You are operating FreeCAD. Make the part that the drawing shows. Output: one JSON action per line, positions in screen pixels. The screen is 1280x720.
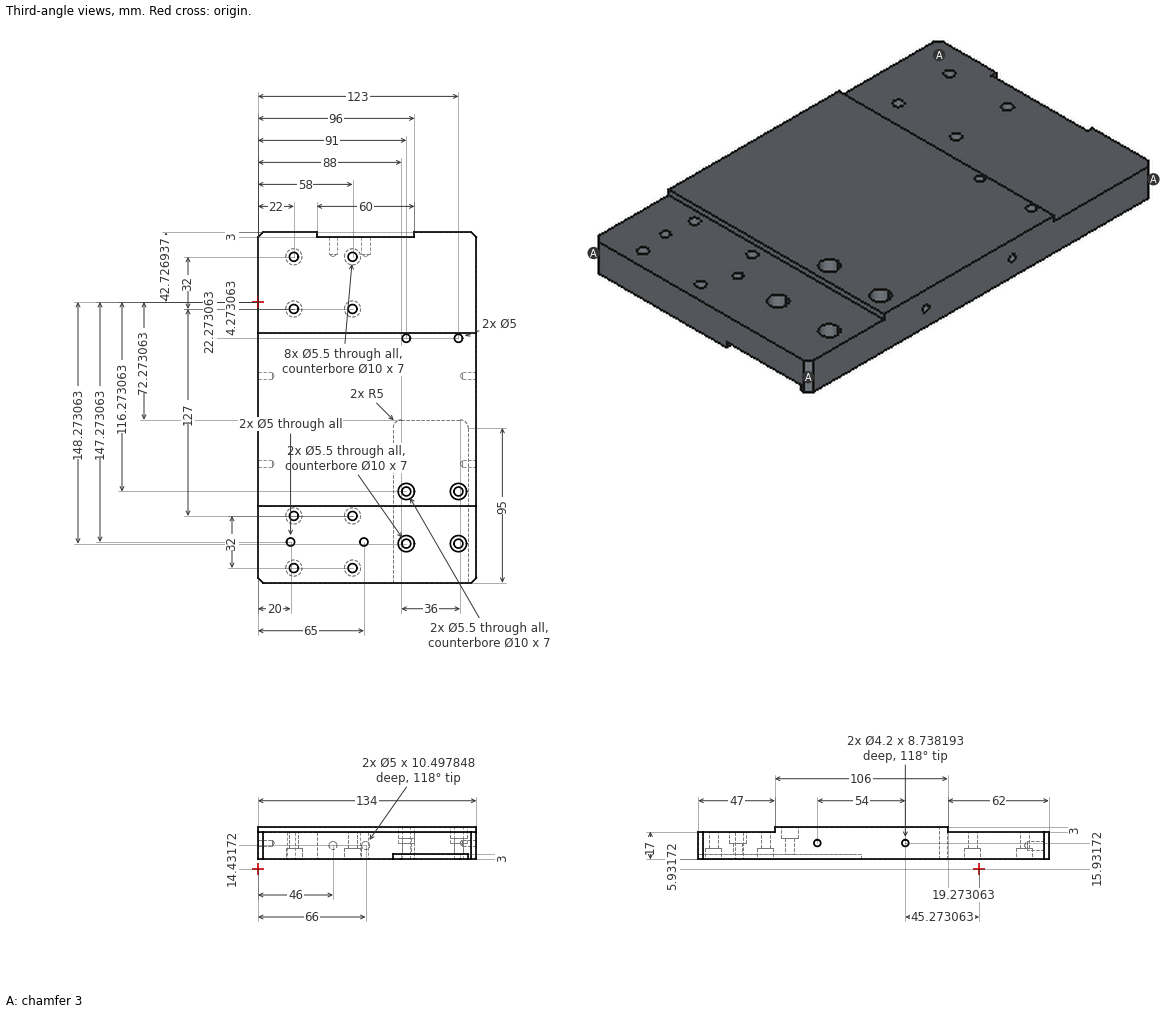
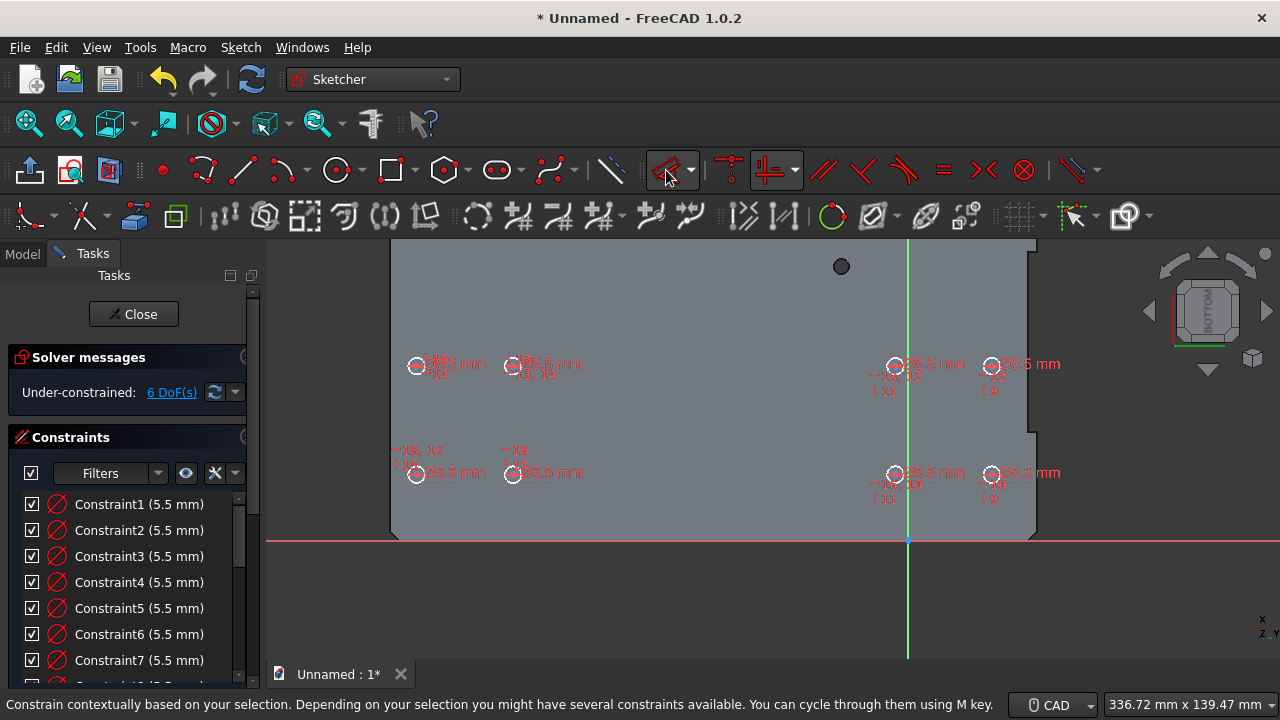
{"action": "left_click", "coordinate": [992, 366]}
{"action": "left_click", "coordinate": [1026, 453]}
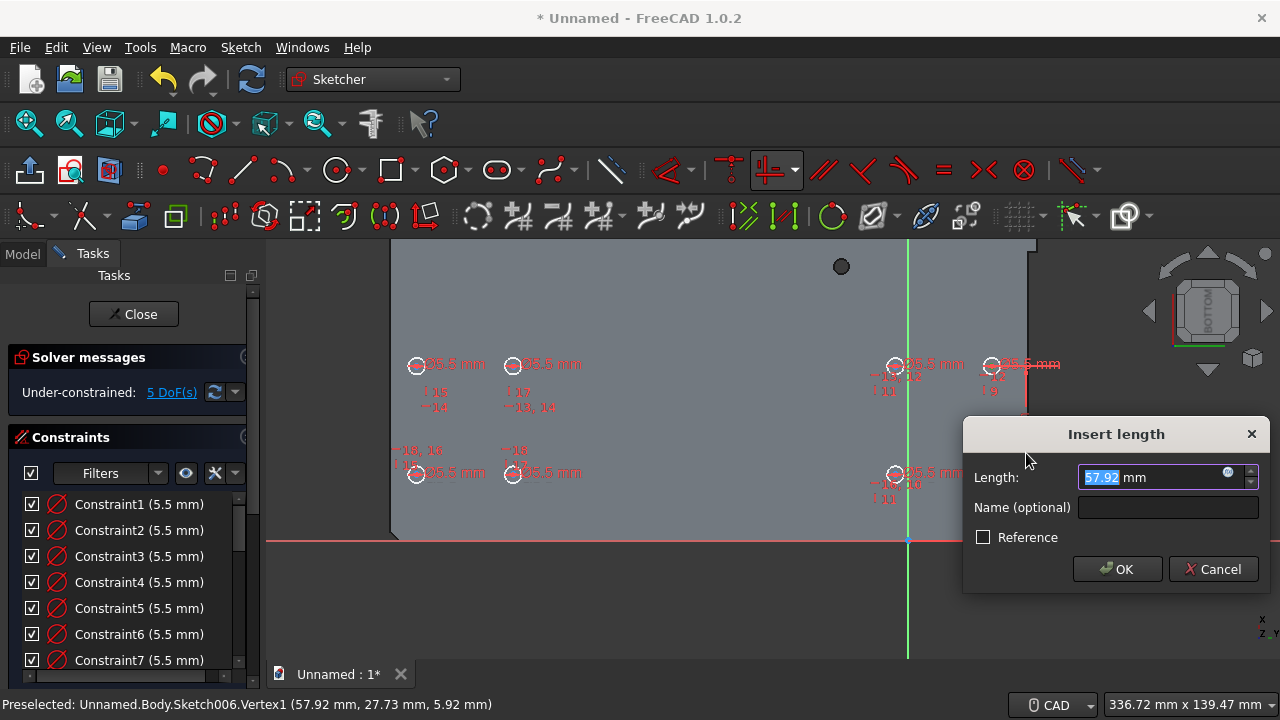
{"action": "type", "text": "58"}
{"action": "key", "text": "Return"}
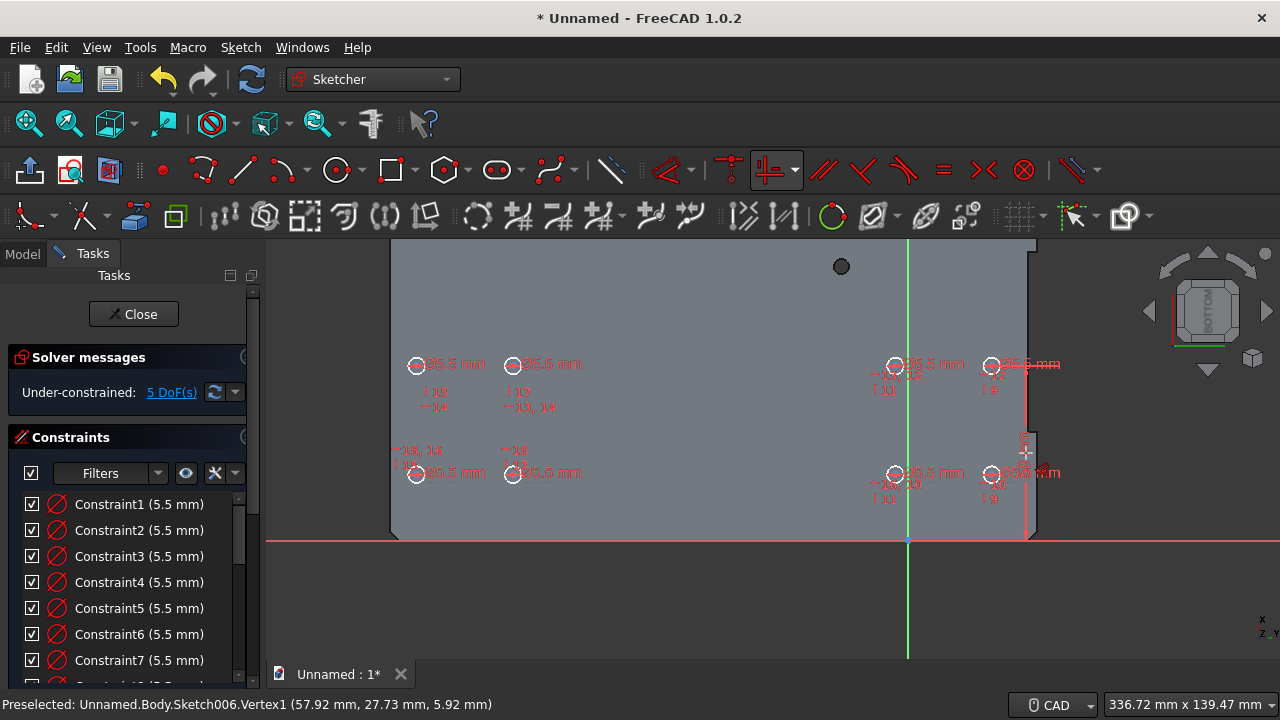
{"action": "left_click", "coordinate": [992, 475]}
{"action": "left_click", "coordinate": [1026, 508]}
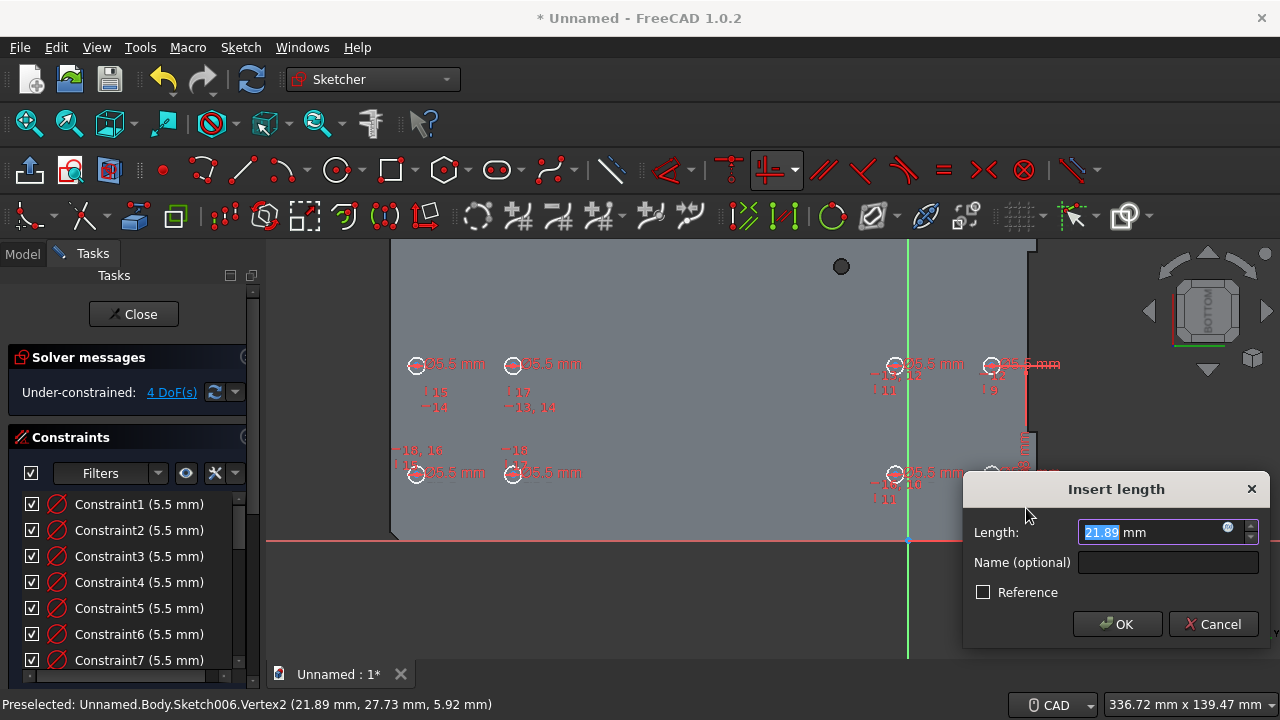
{"action": "type", "text": "22"}
{"action": "key", "text": "Return"}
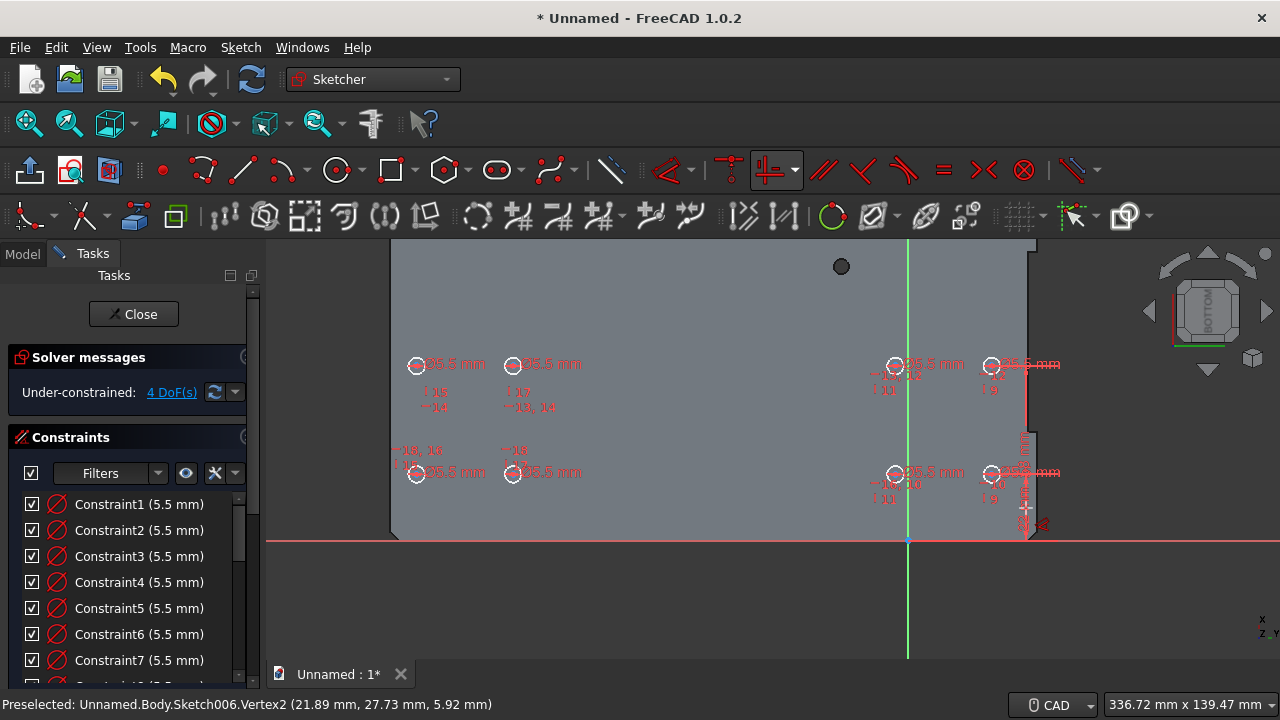
{"action": "left_click", "coordinate": [992, 474]}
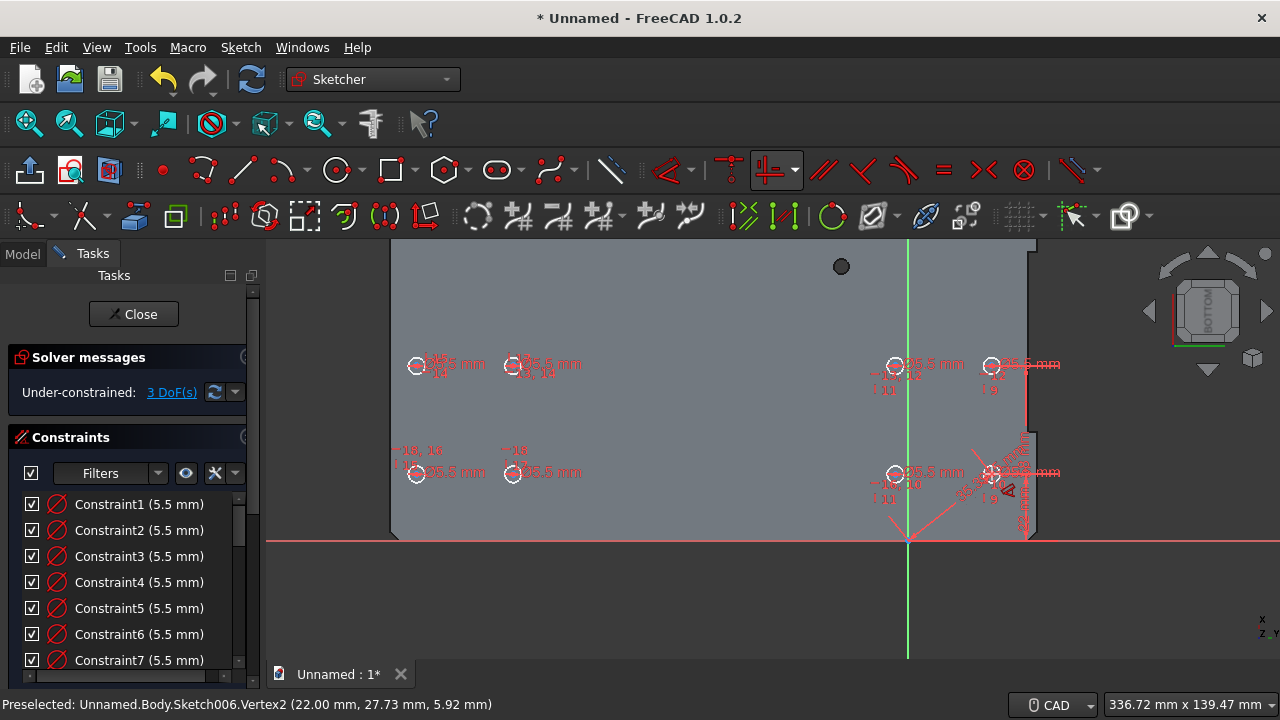
{"action": "left_click", "coordinate": [896, 474]}
{"action": "left_click", "coordinate": [944, 508]}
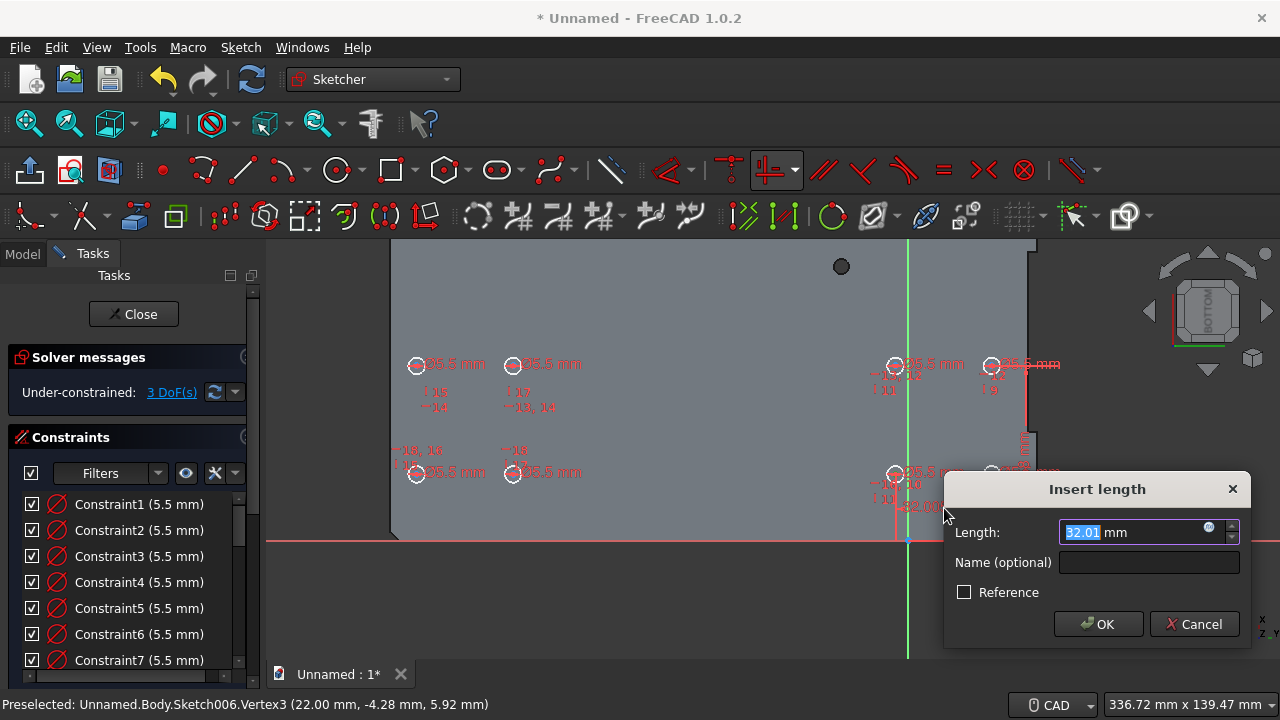
{"action": "type", "text": "32"}
{"action": "key", "text": "Return"}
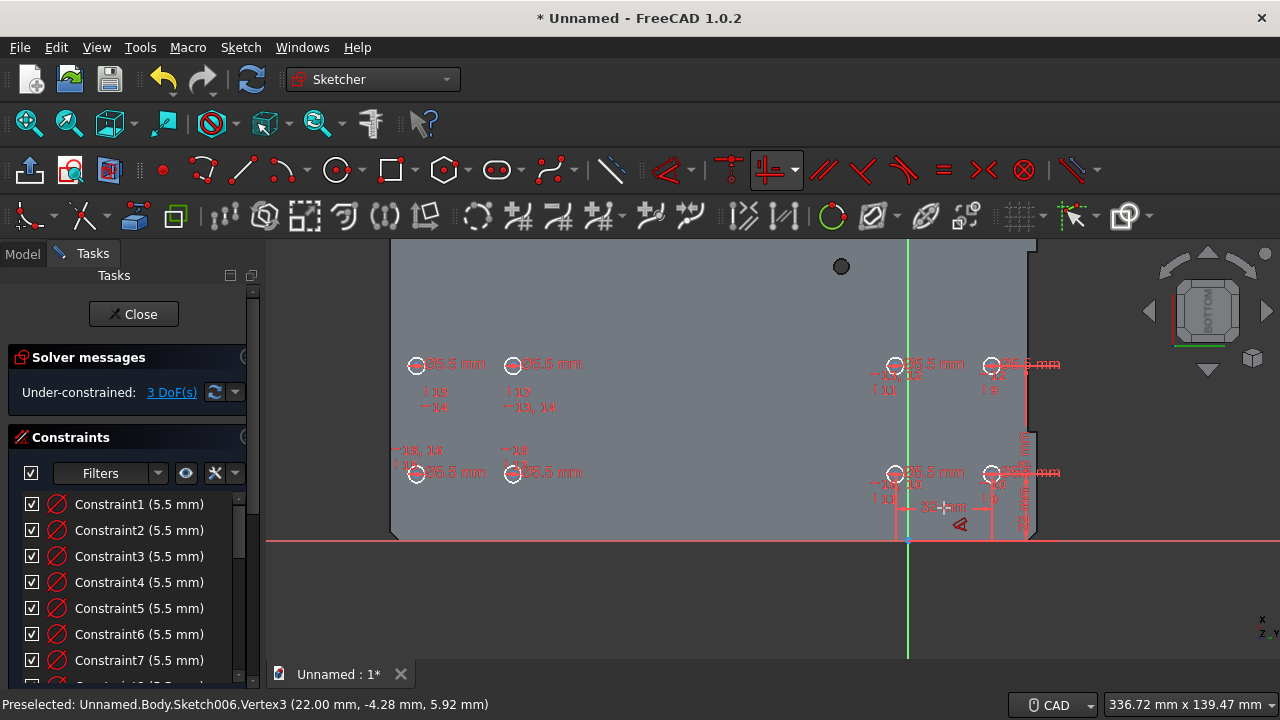
{"action": "left_click", "coordinate": [513, 366]}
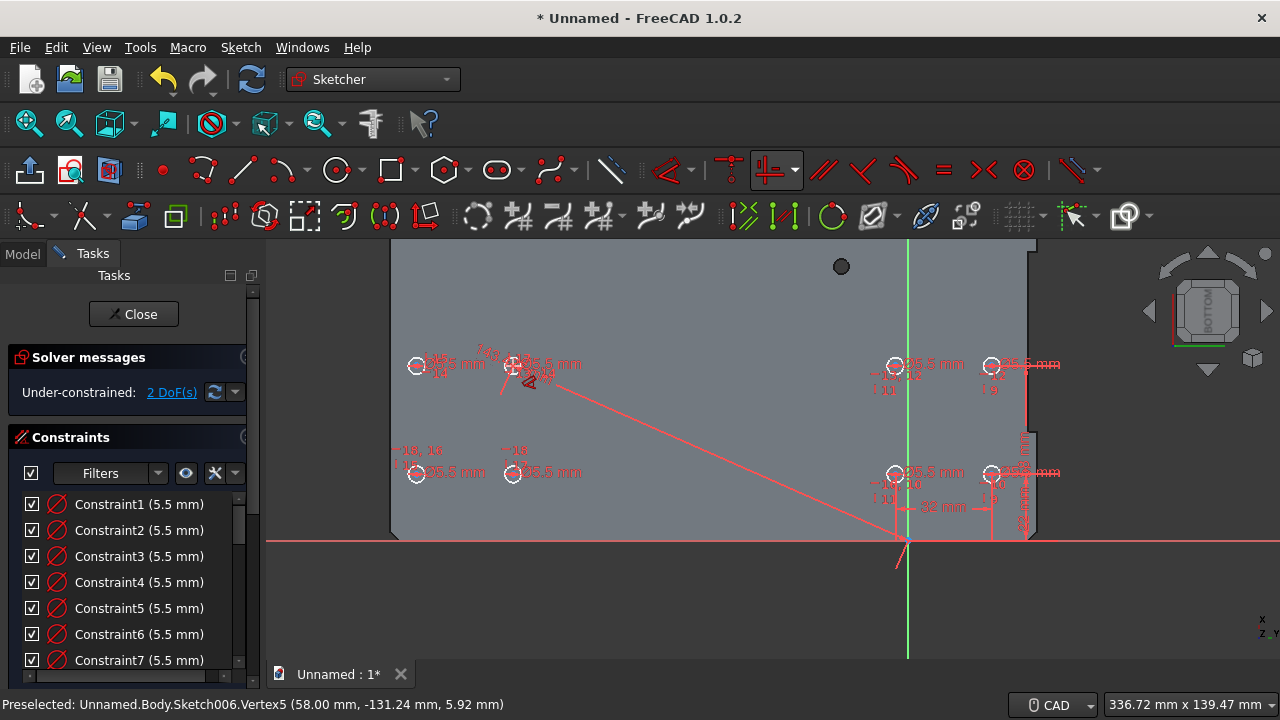
{"action": "left_click", "coordinate": [417, 366]}
{"action": "left_click", "coordinate": [465, 332]}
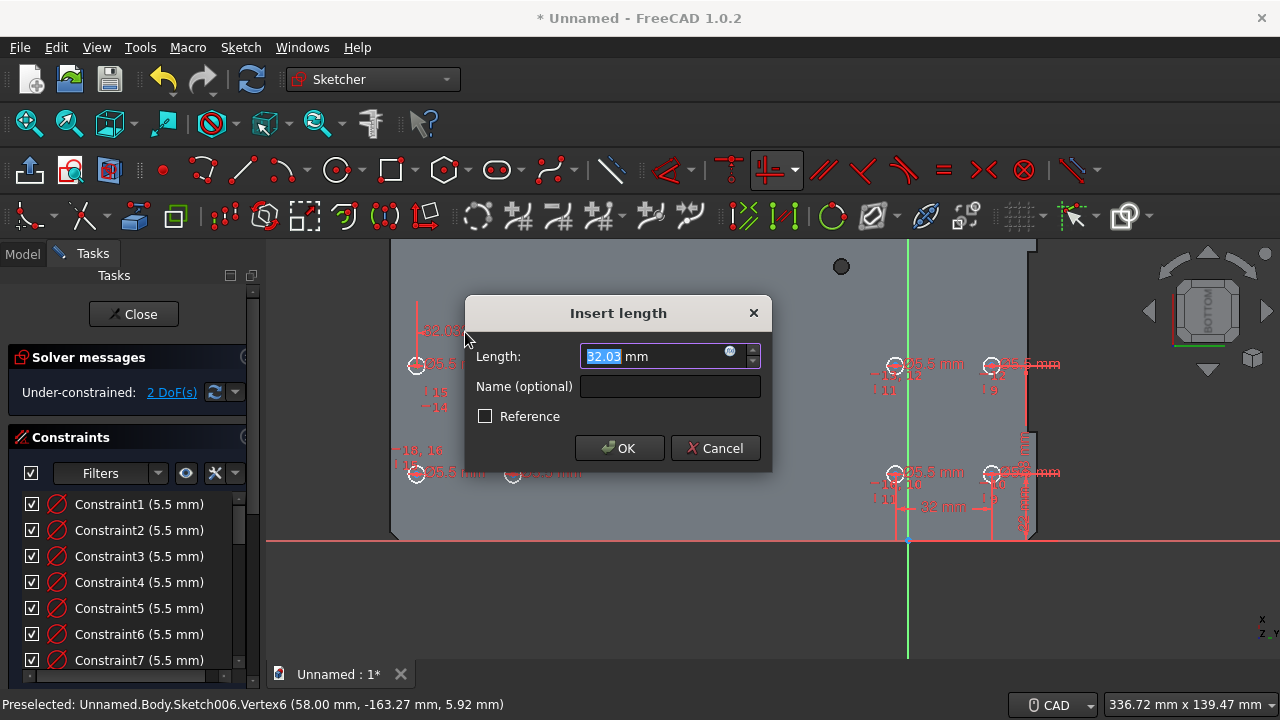
{"action": "type", "text": "32"}
{"action": "key", "text": "Return"}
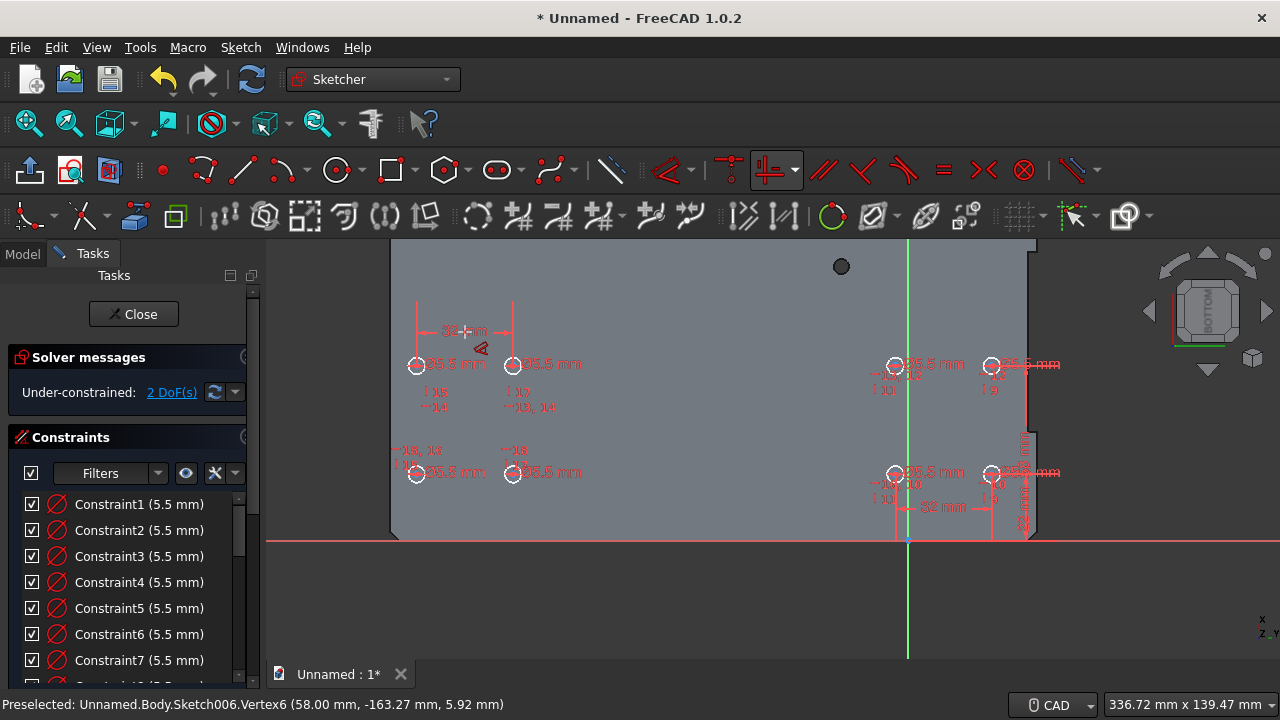
{"action": "left_click", "coordinate": [896, 366]}